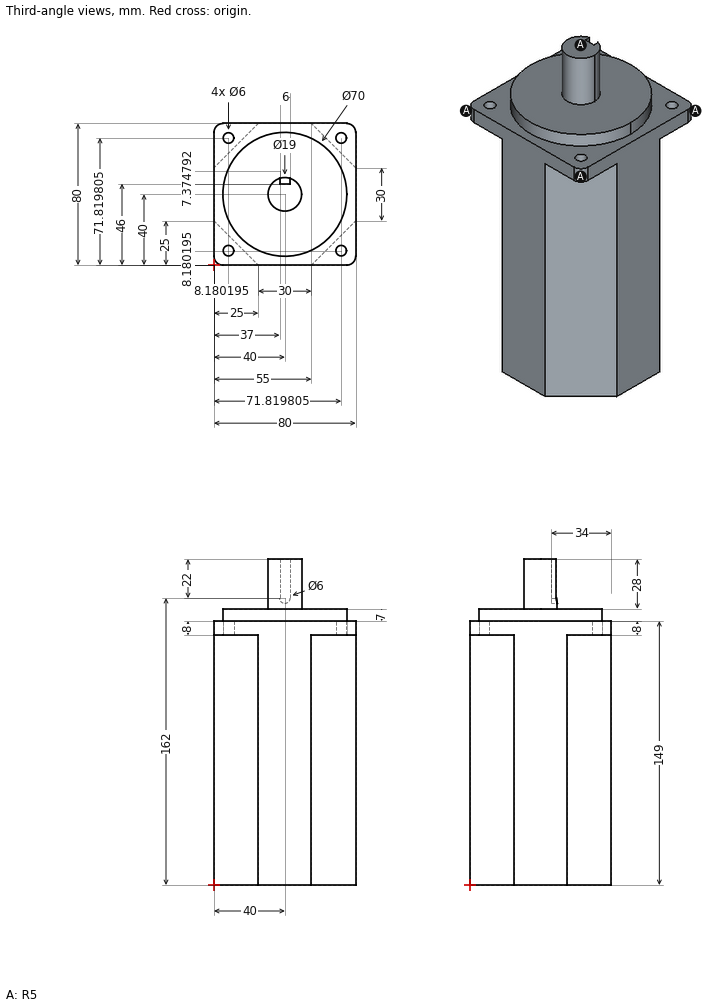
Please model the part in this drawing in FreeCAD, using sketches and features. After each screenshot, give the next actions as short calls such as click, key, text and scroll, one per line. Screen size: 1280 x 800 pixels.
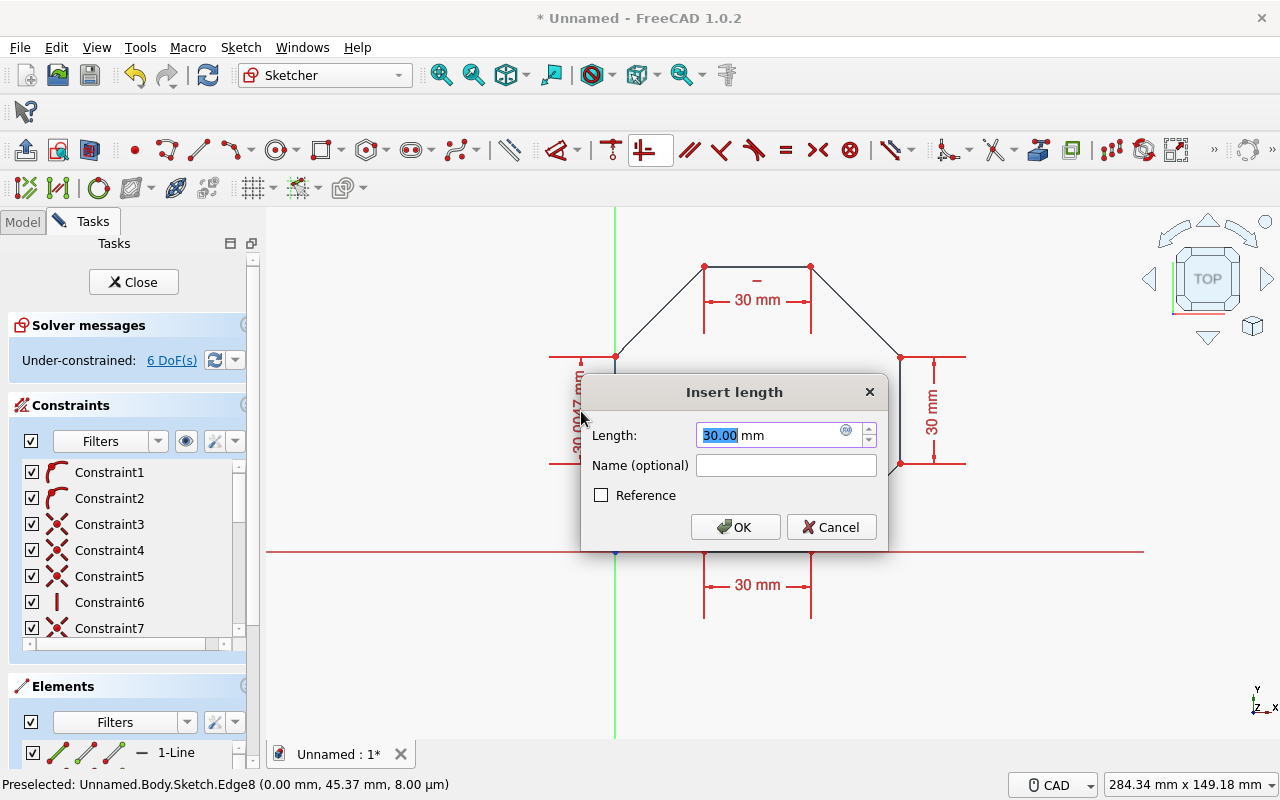
text(30)
key(Return)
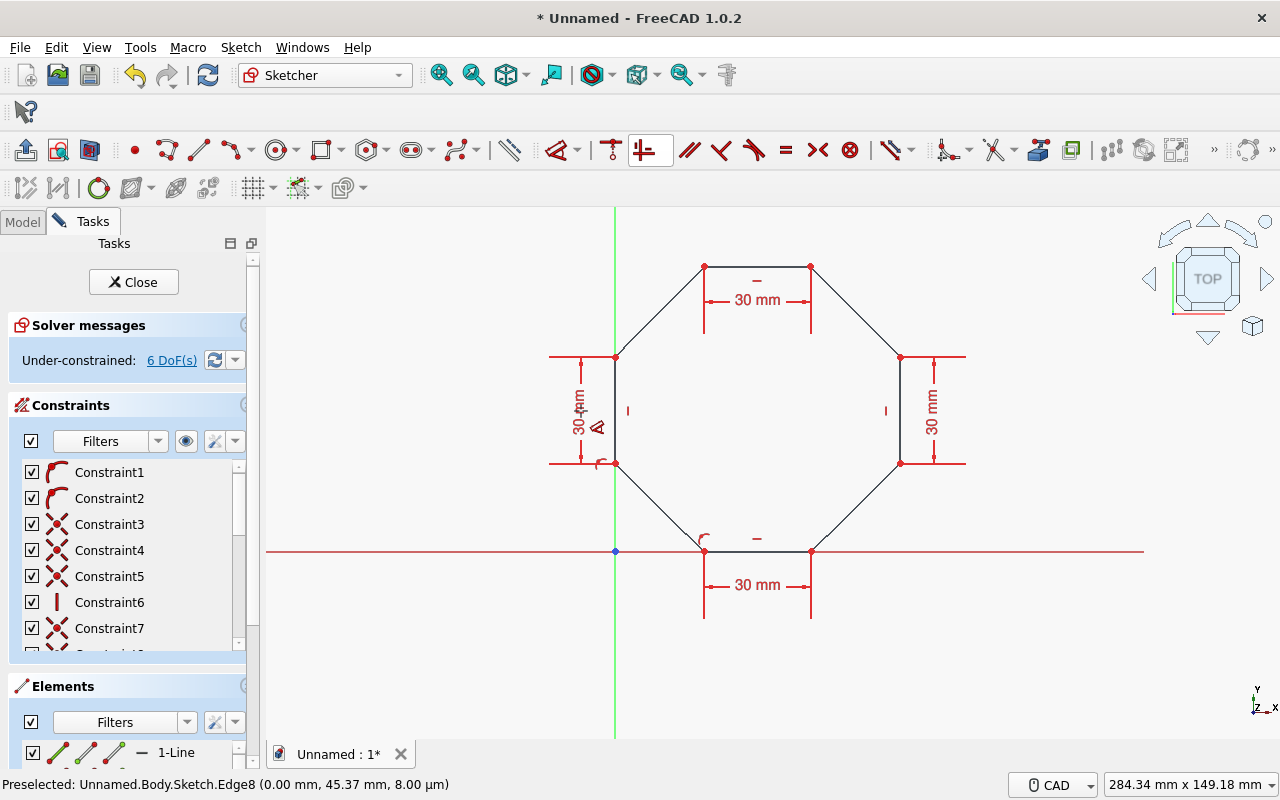
click(615, 464)
click(581, 508)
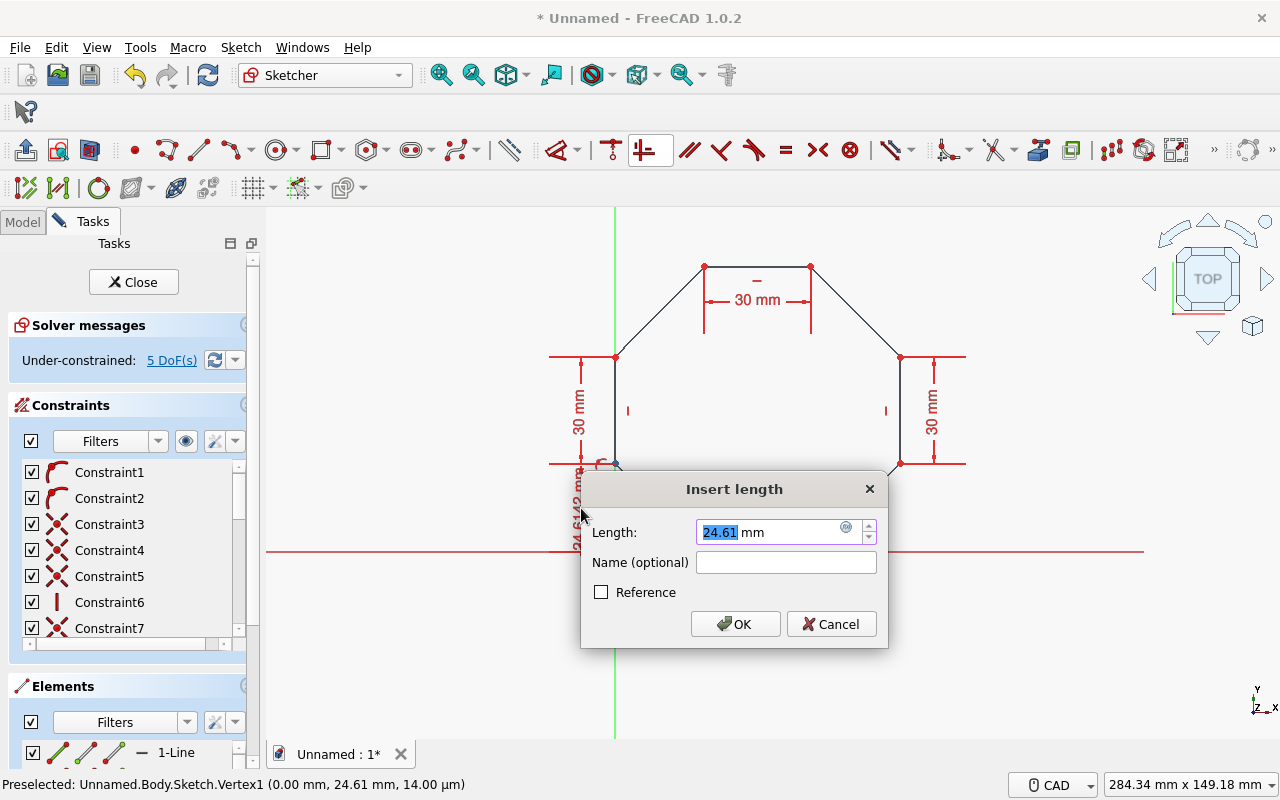
text(25)
key(Return)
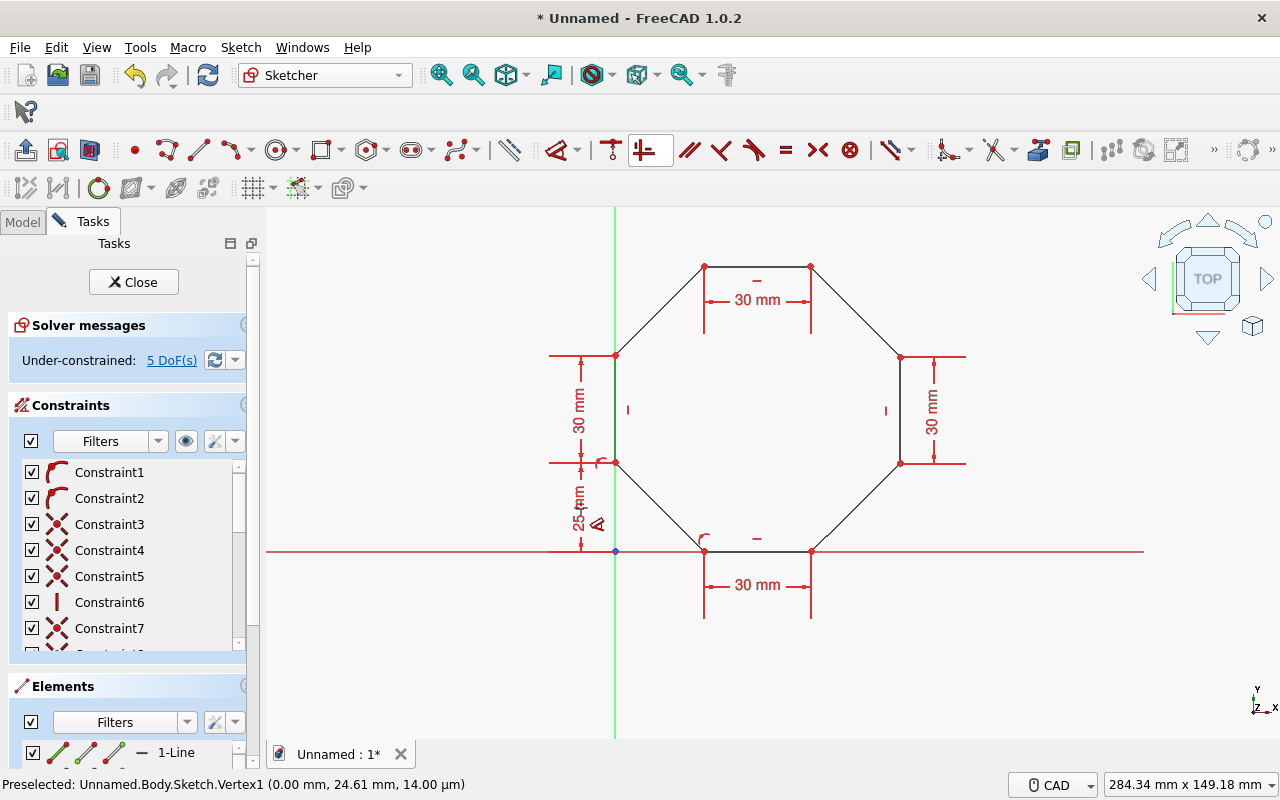
click(704, 552)
click(660, 586)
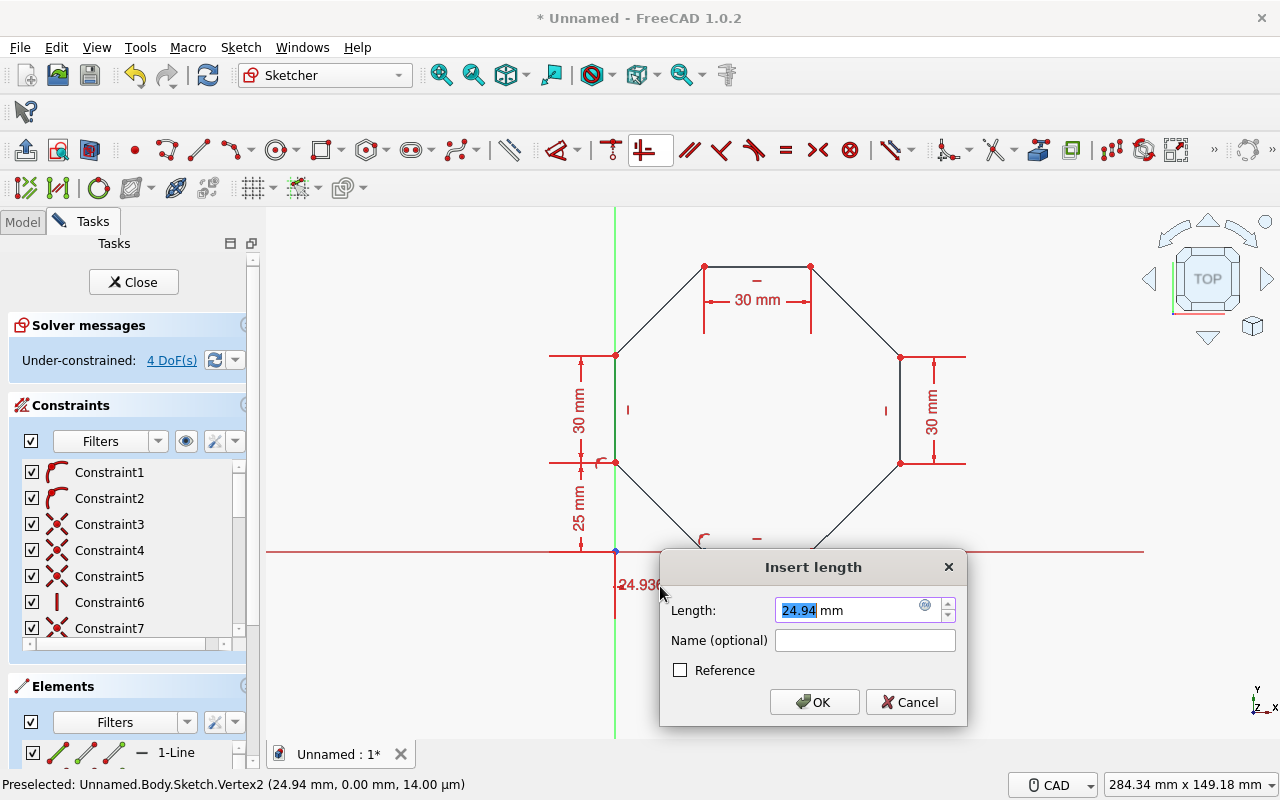
text(25)
key(Return)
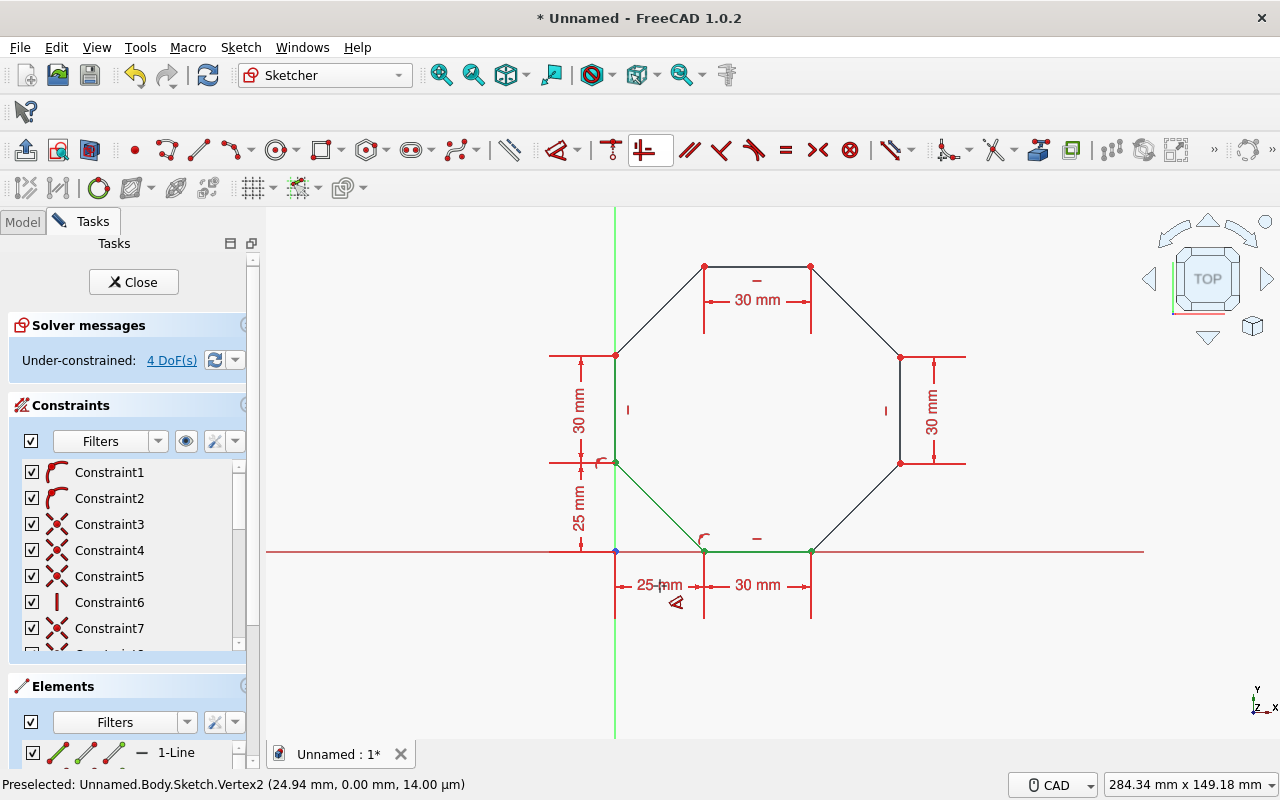
click(900, 464)
click(857, 586)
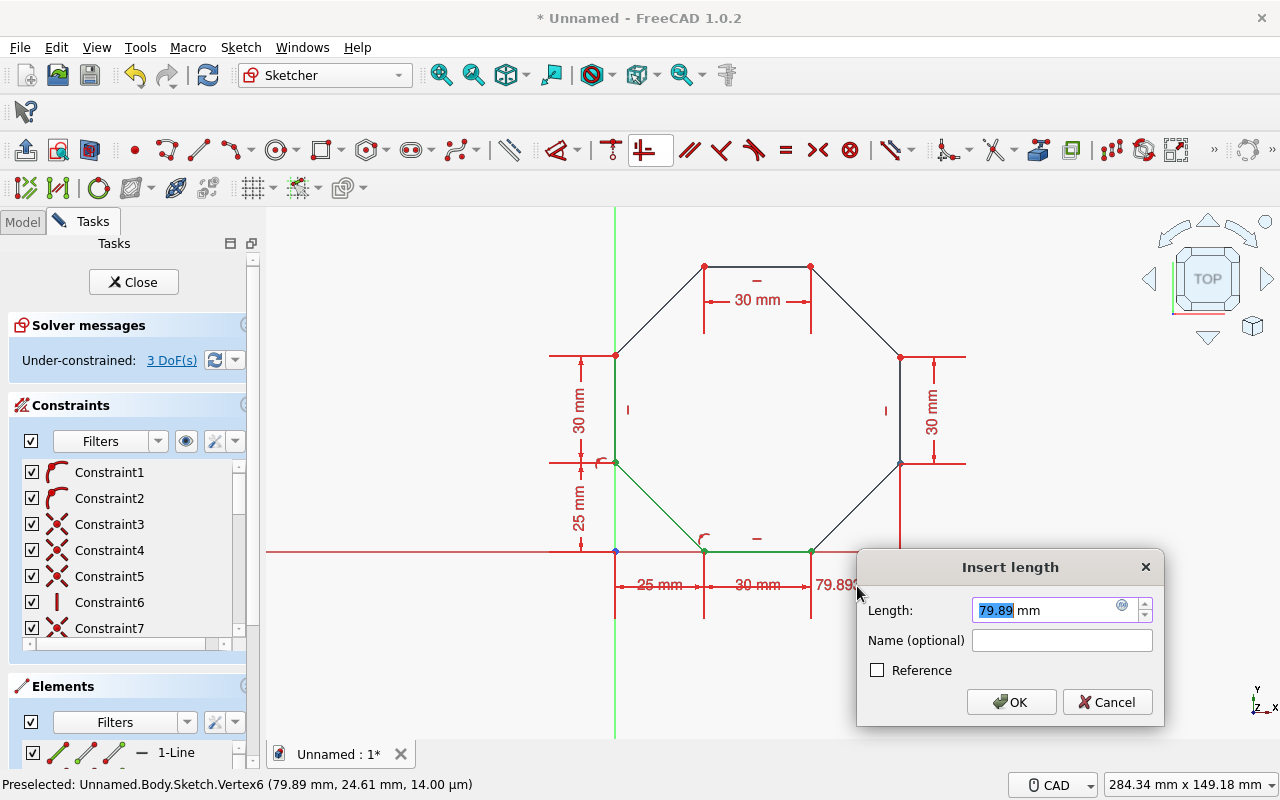
text(80)
key(Return)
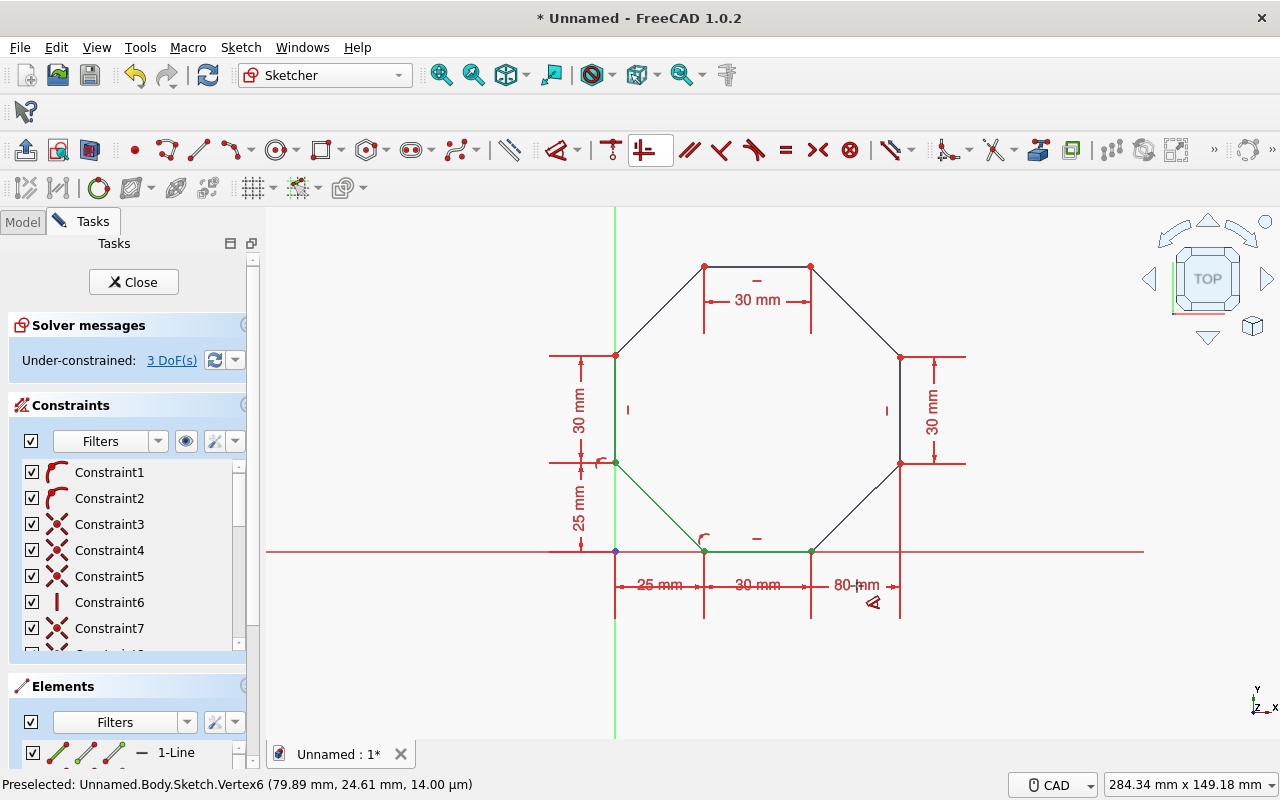
click(900, 464)
click(934, 508)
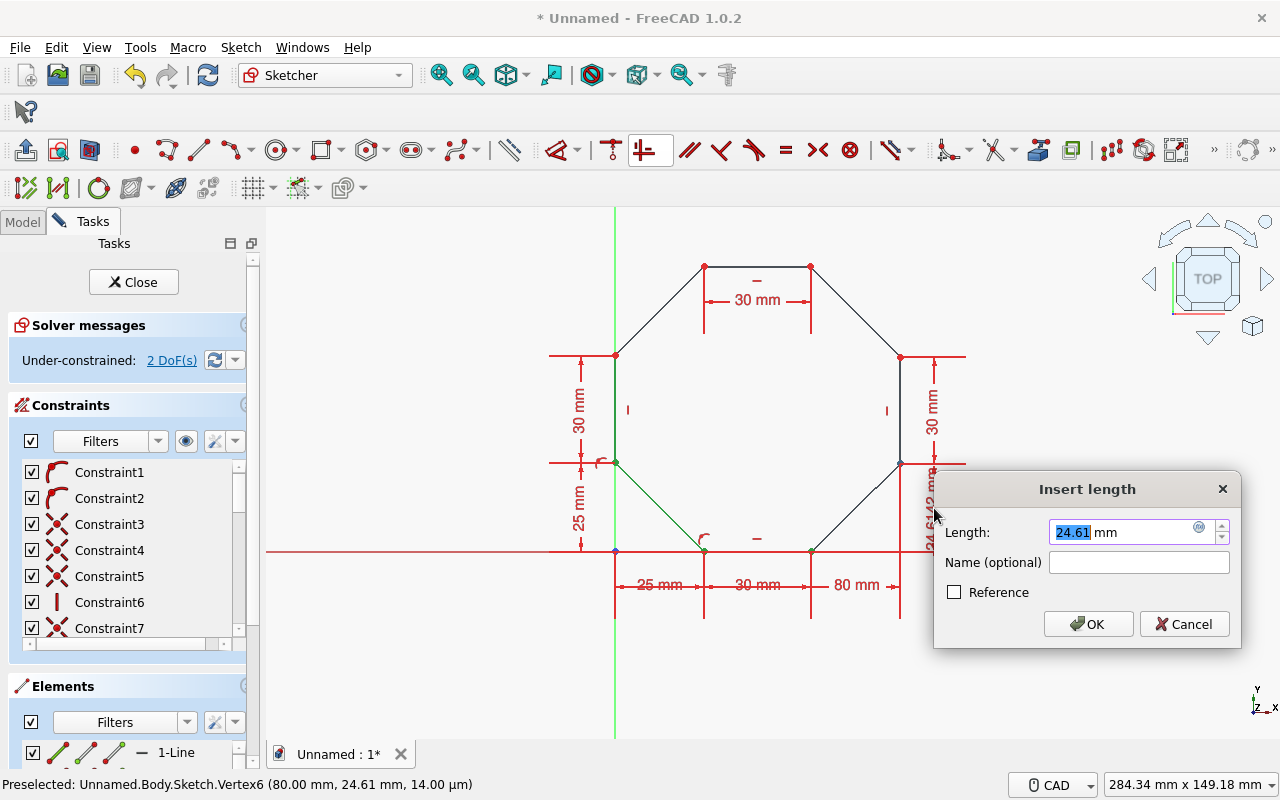
text(25)
key(Return)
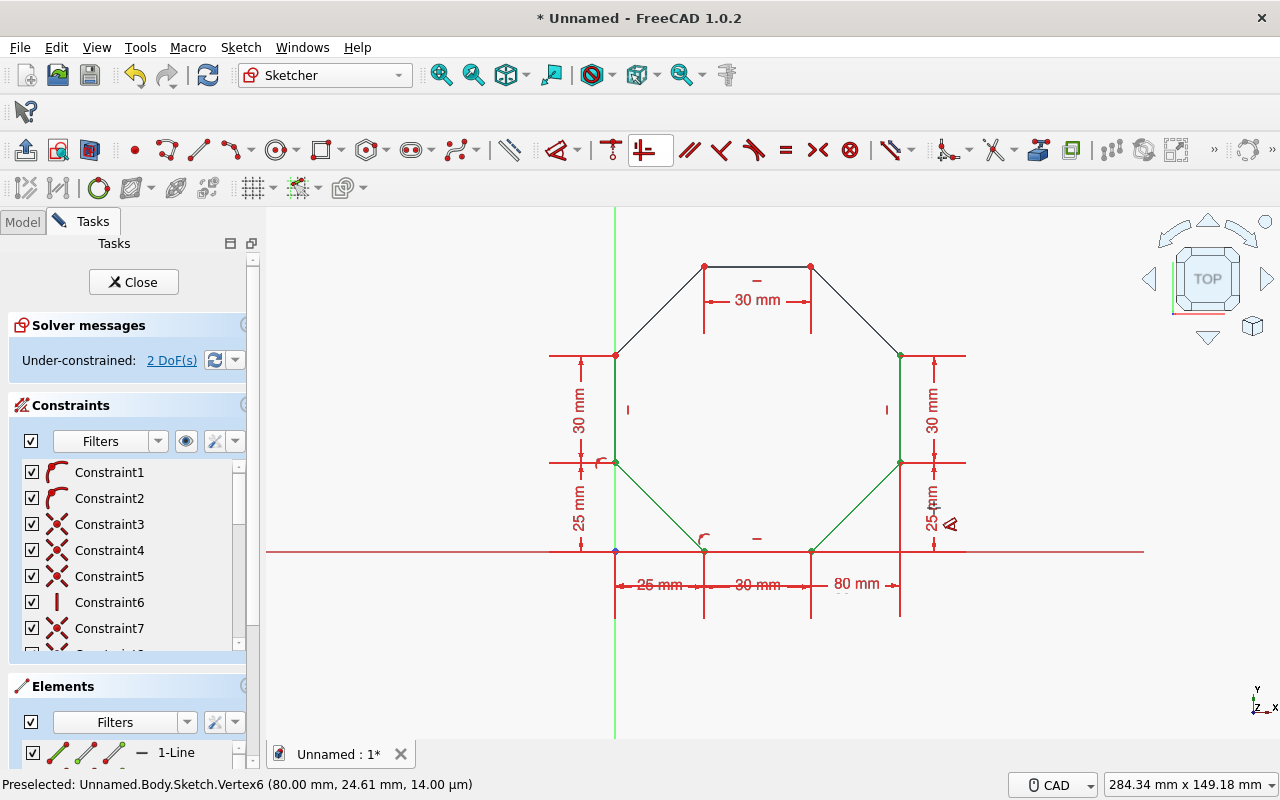
click(811, 267)
click(713, 610)